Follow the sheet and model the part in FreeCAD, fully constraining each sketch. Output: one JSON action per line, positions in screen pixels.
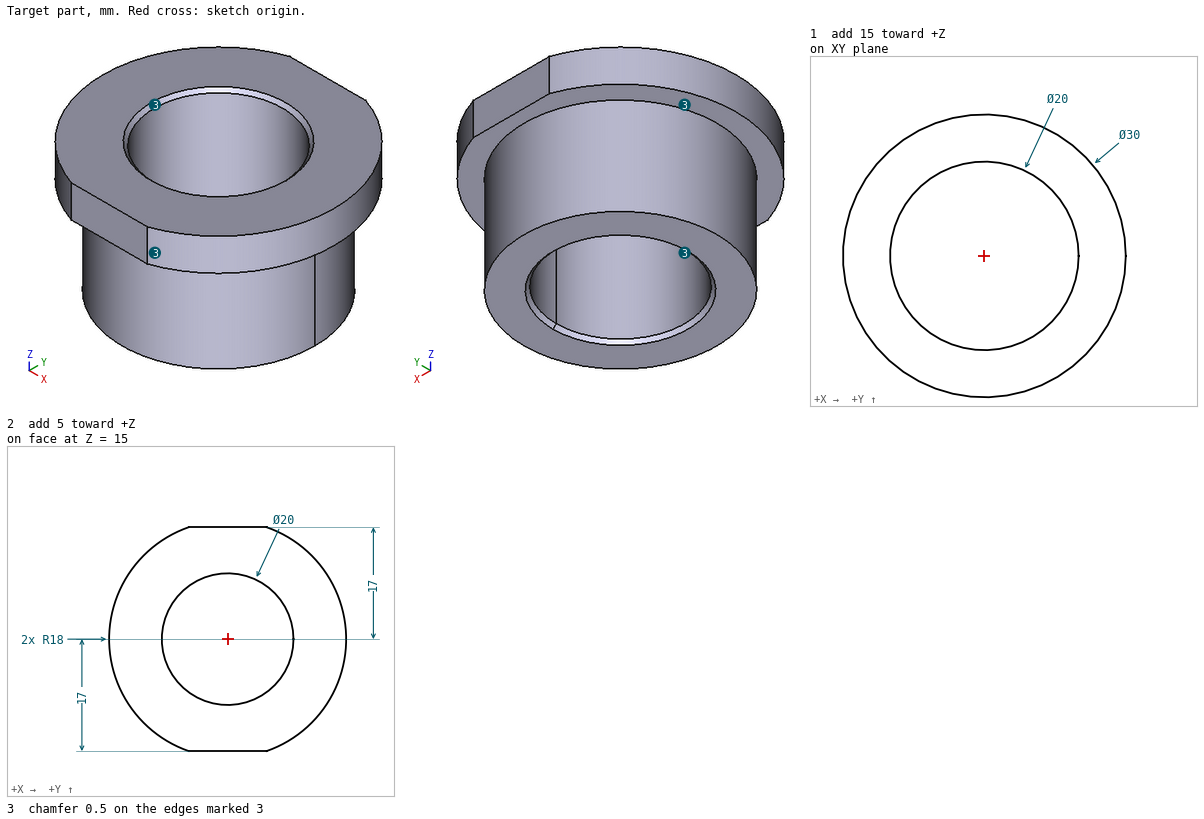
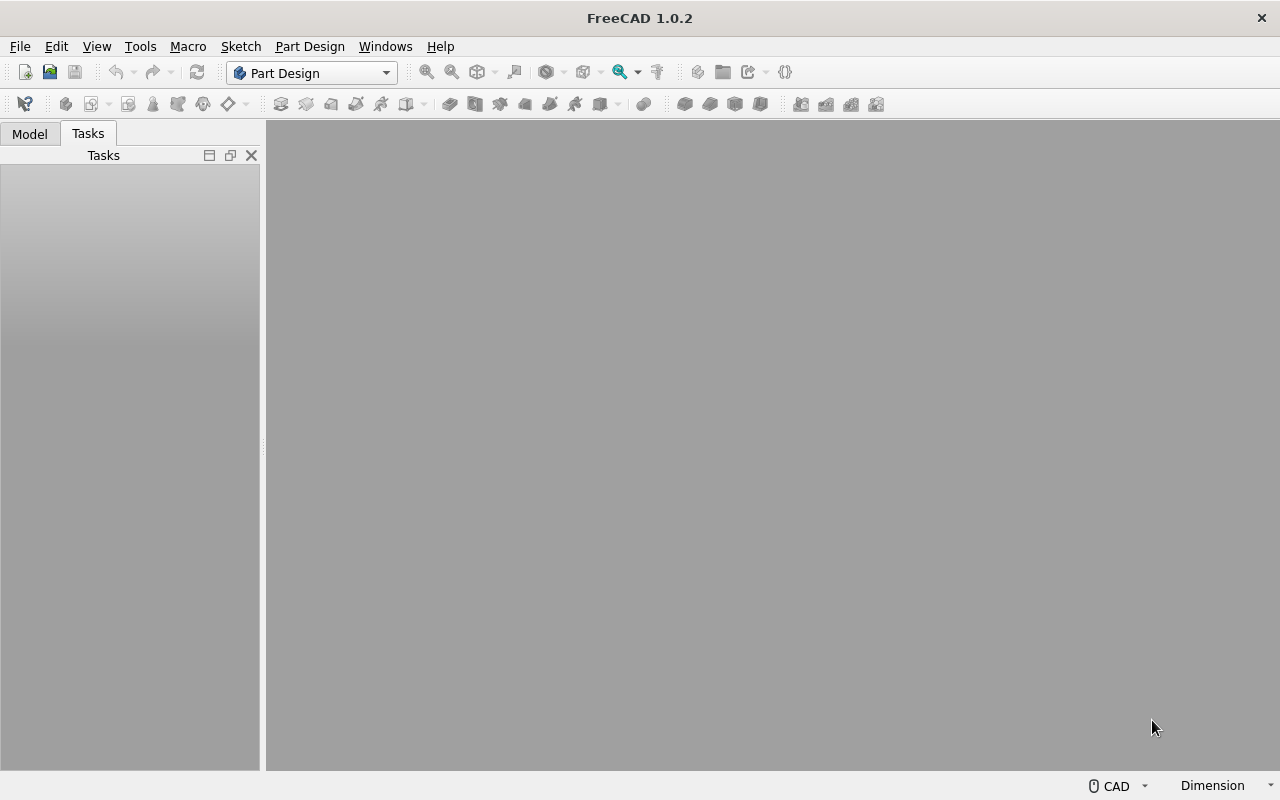
{"action": "left_click", "coordinate": [25, 72]}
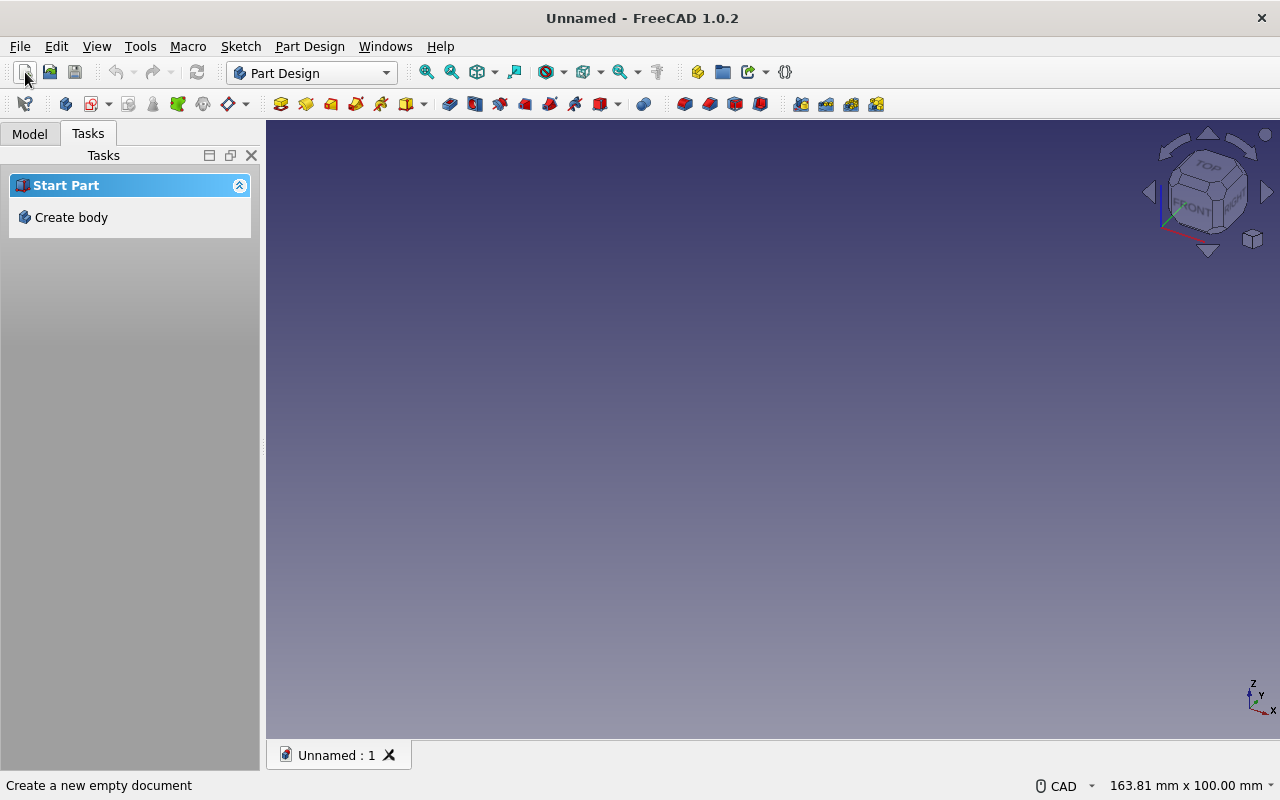
{"action": "left_click", "coordinate": [90, 104]}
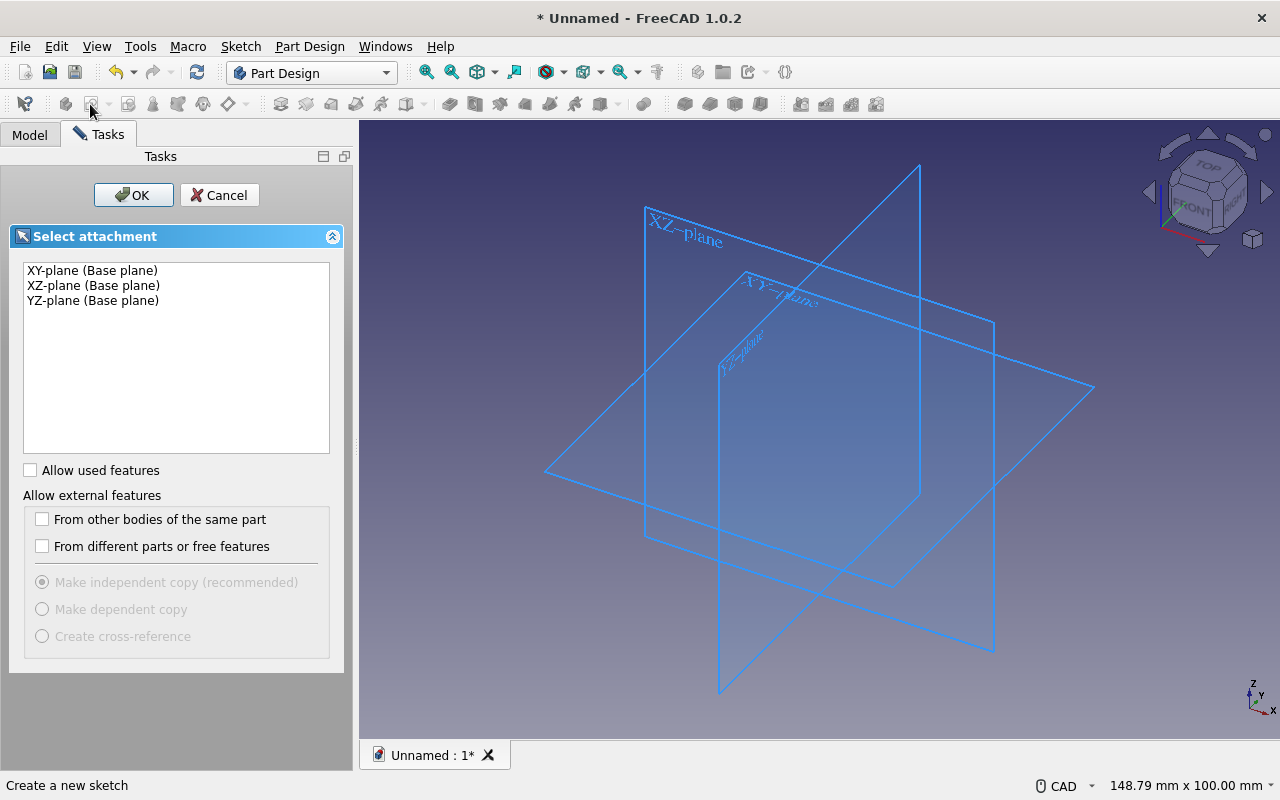
{"action": "left_click", "coordinate": [84, 270]}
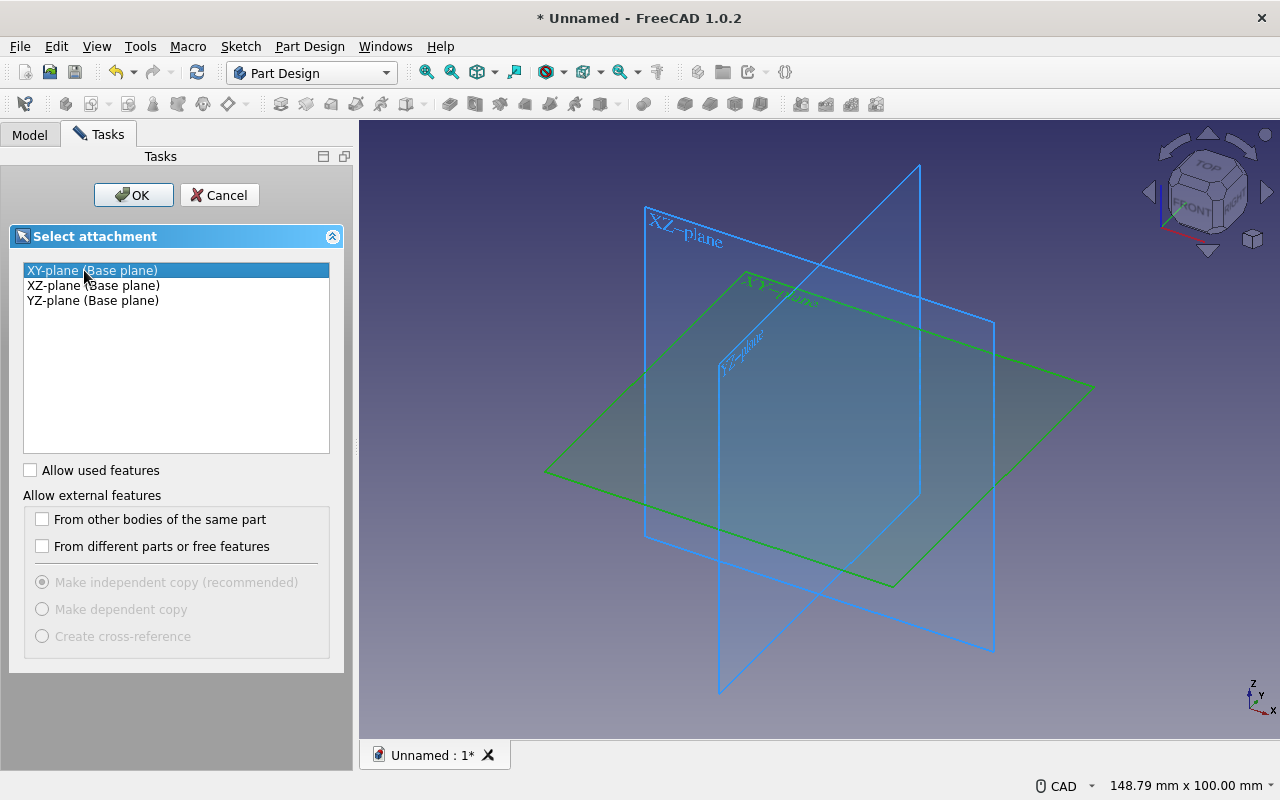
{"action": "left_click", "coordinate": [134, 195]}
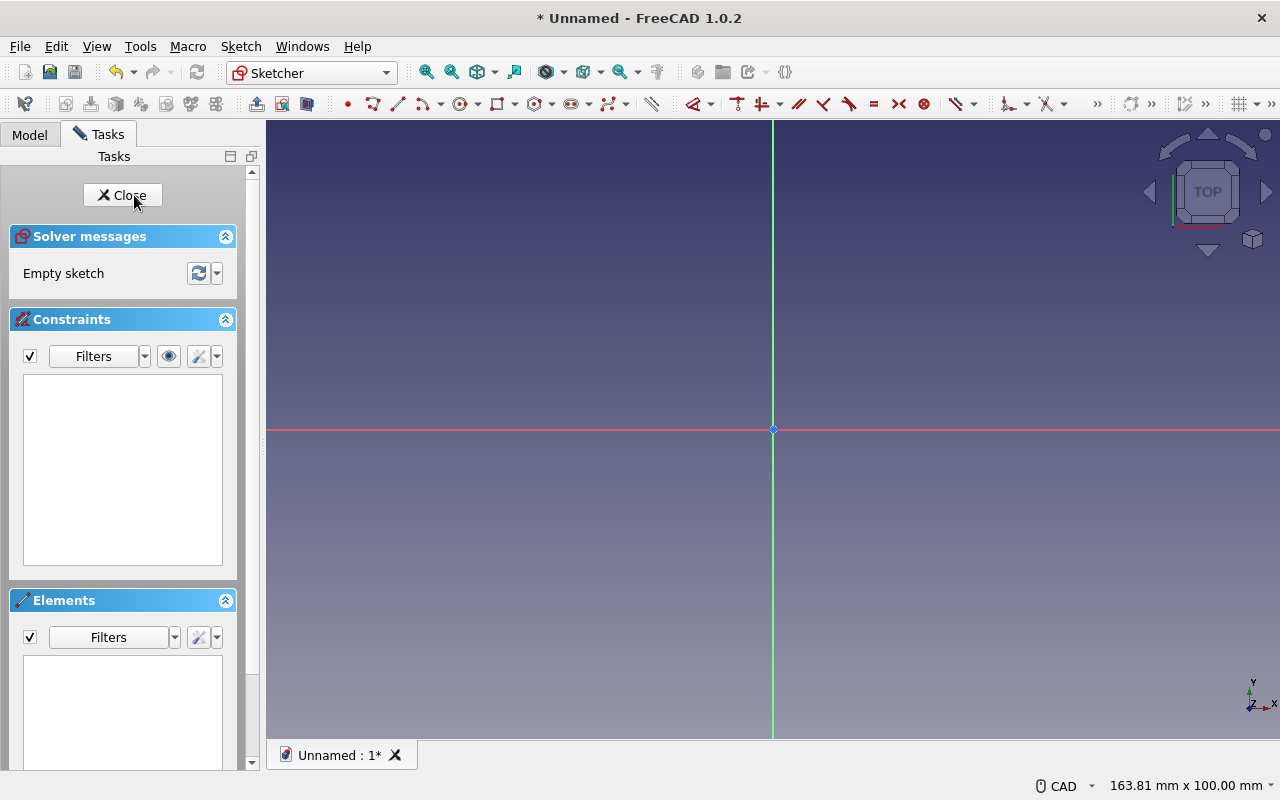
{"action": "scroll", "coordinate": [829, 430], "scroll_direction": "up", "scroll_amount": 4}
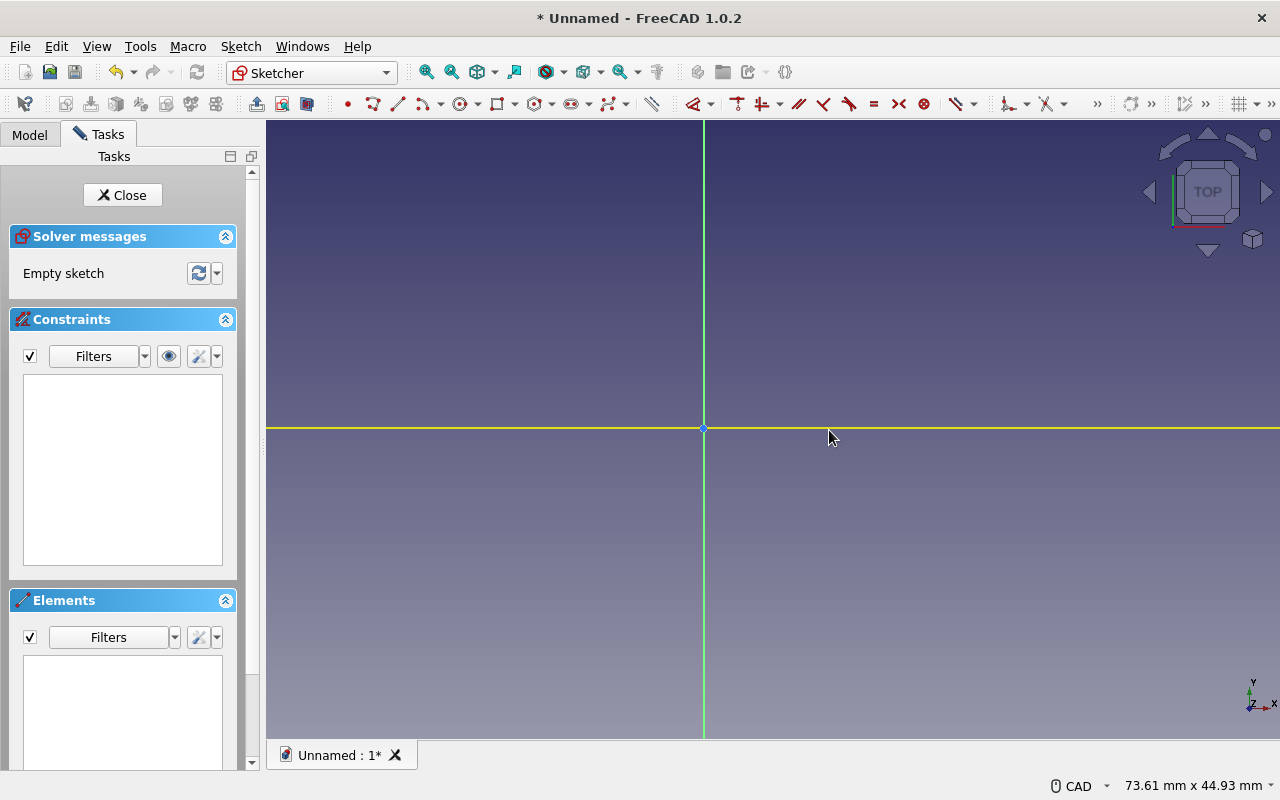
{"action": "left_click", "coordinate": [460, 104]}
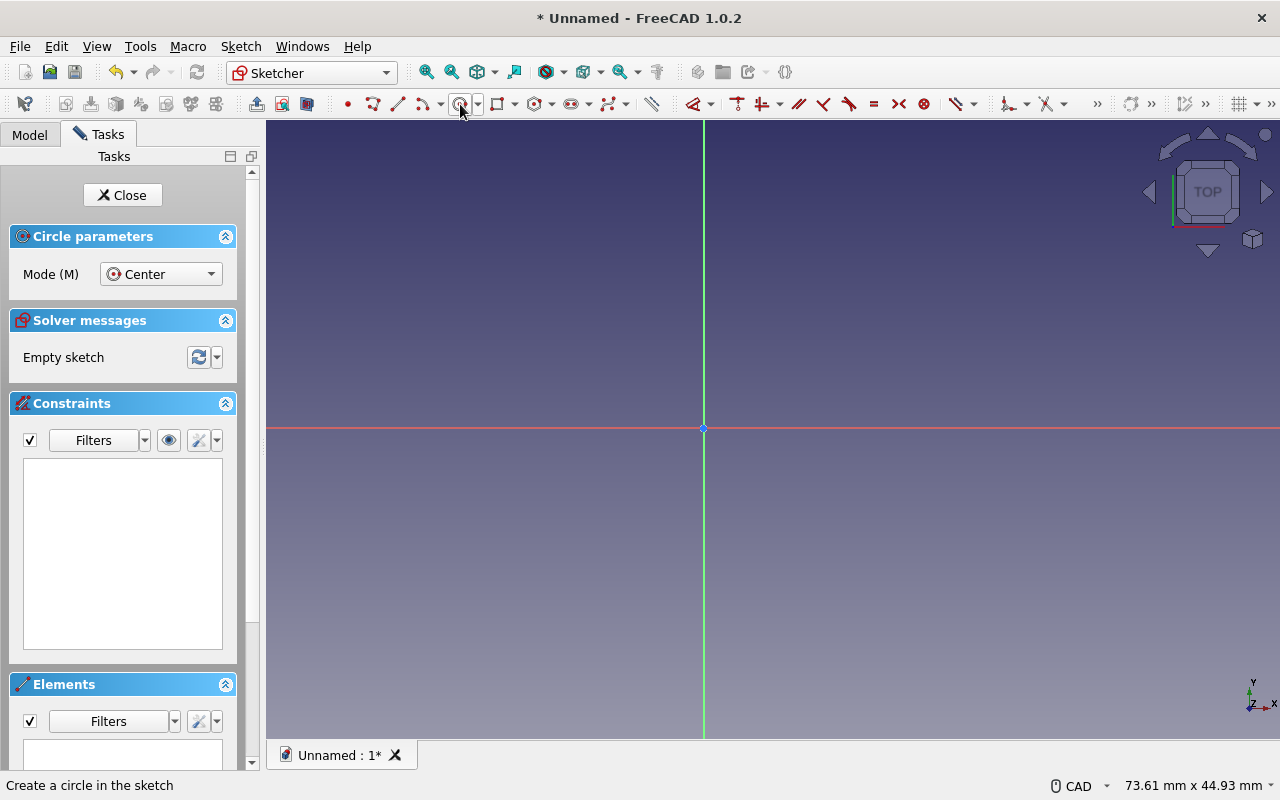
{"action": "left_click", "coordinate": [704, 428]}
{"action": "mouse_move", "coordinate": [850, 282]}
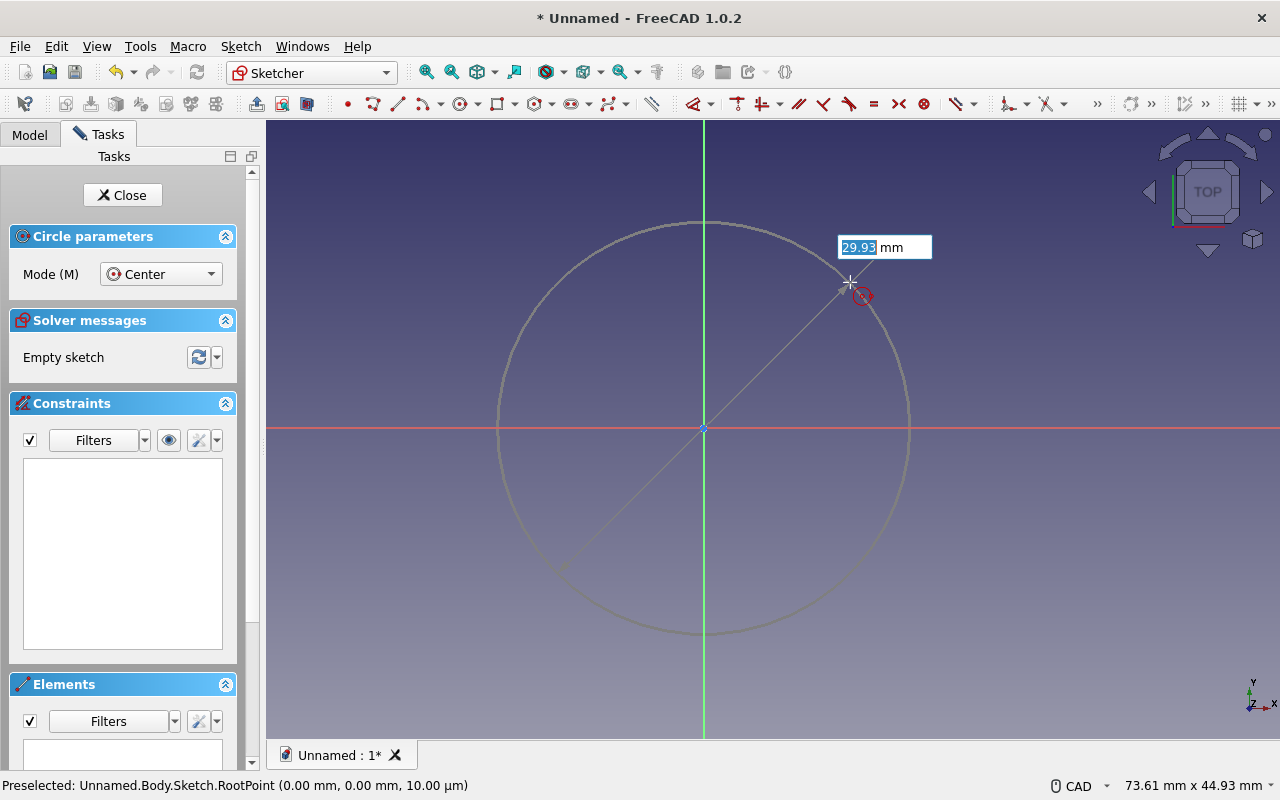
{"action": "type", "text": "30"}
{"action": "key", "text": "Return"}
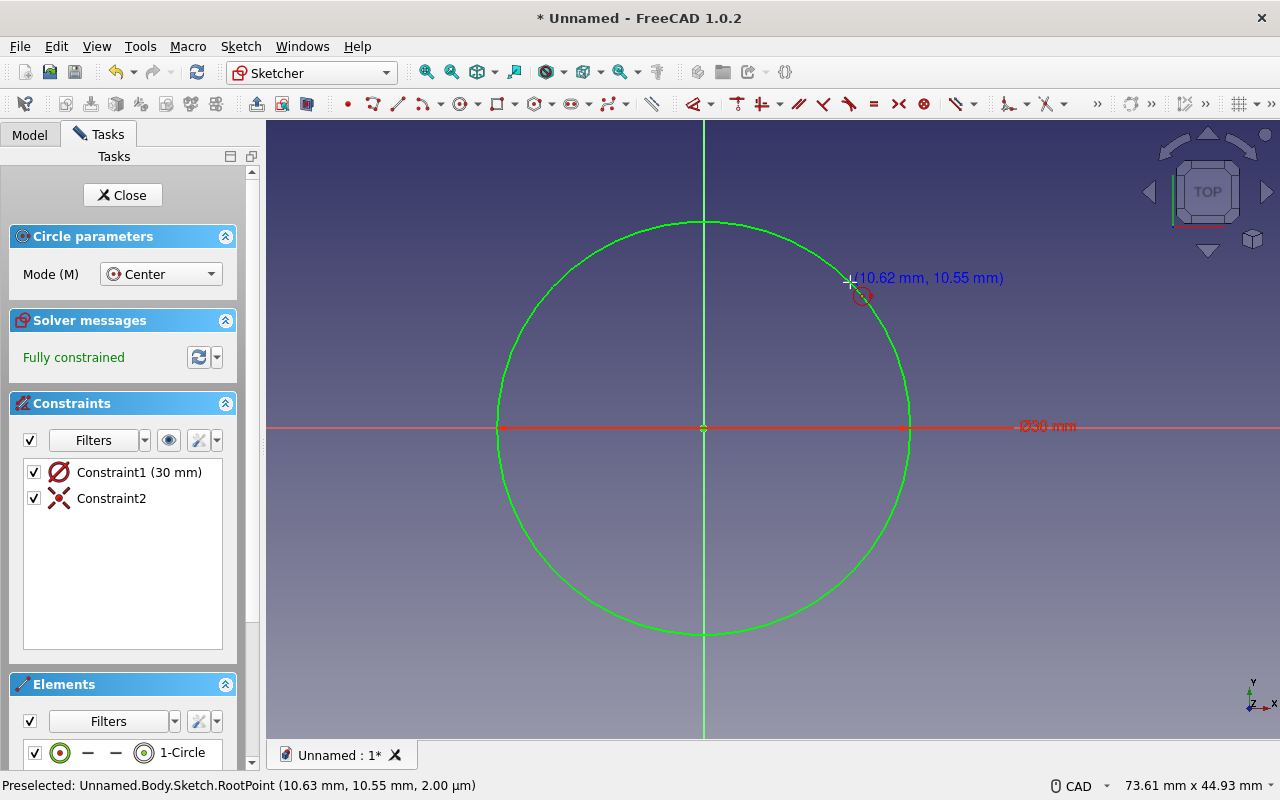
{"action": "left_click", "coordinate": [704, 428]}
{"action": "mouse_move", "coordinate": [801, 331]}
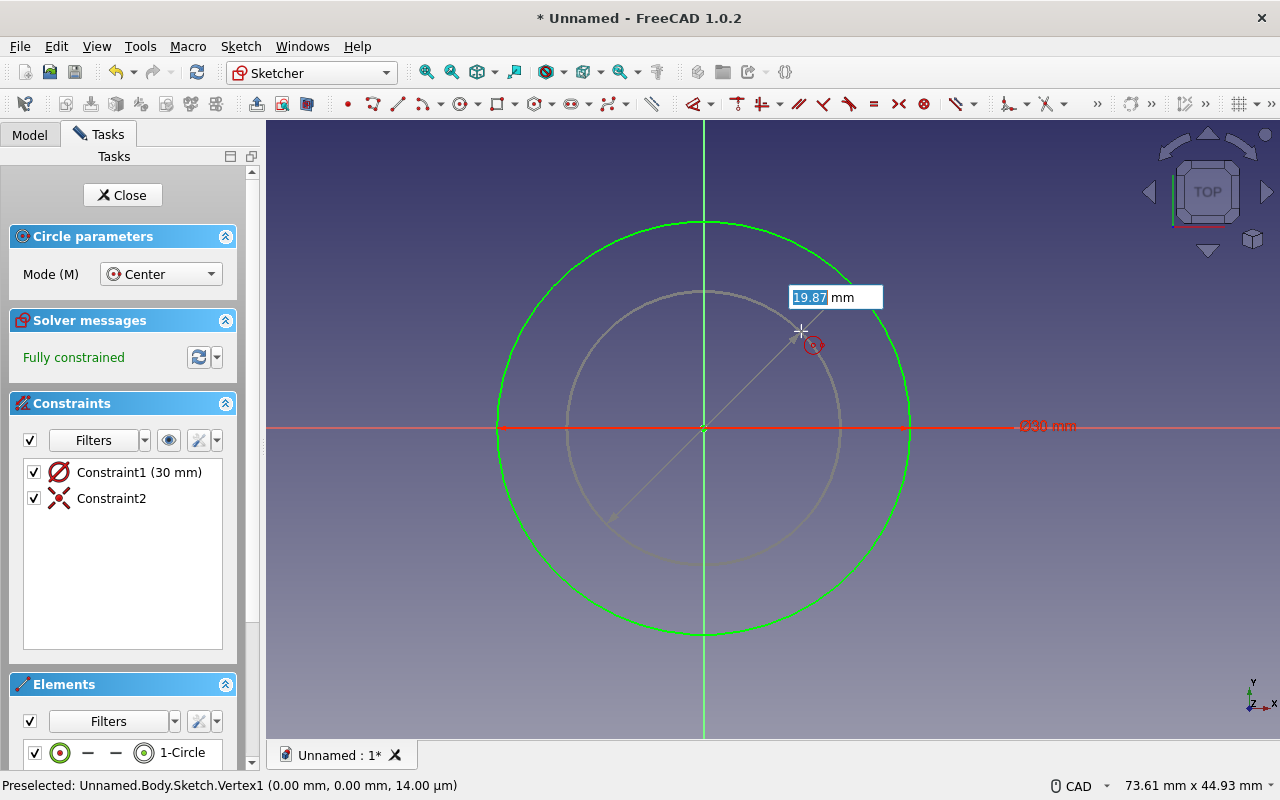
{"action": "type", "text": "20"}
{"action": "key", "text": "Return"}
{"action": "key", "text": "Escape"}